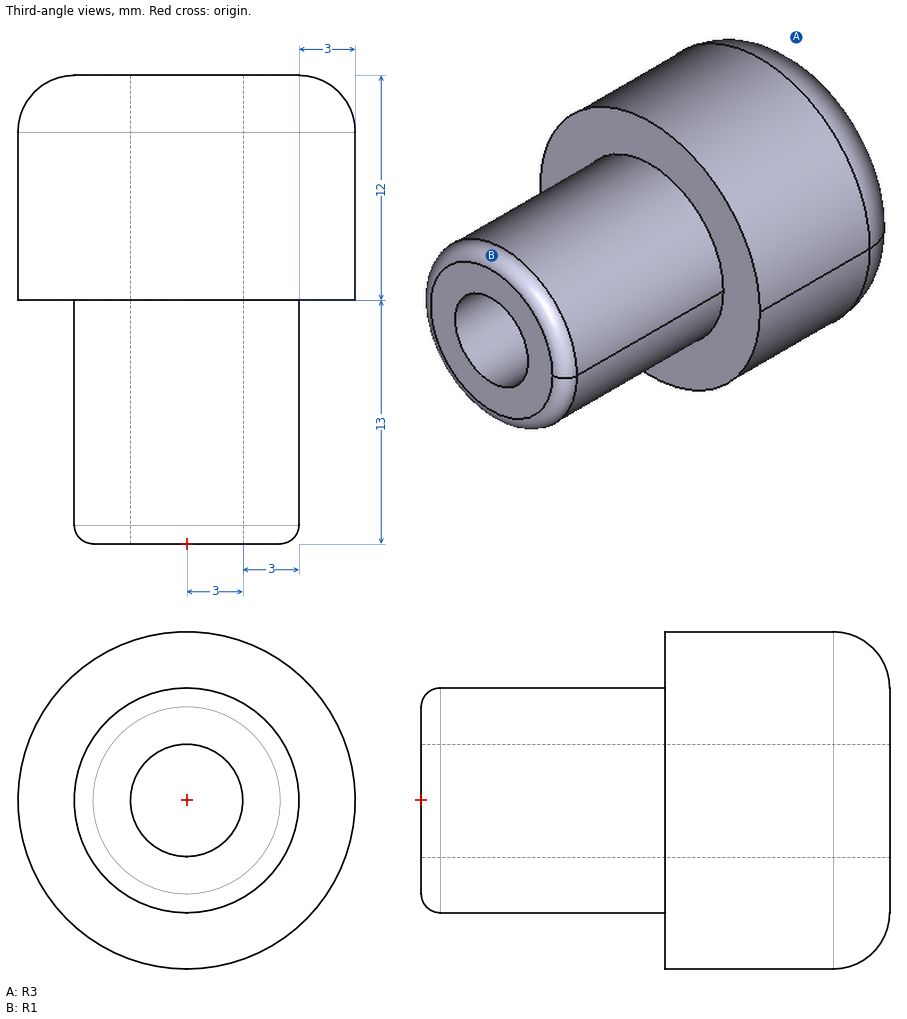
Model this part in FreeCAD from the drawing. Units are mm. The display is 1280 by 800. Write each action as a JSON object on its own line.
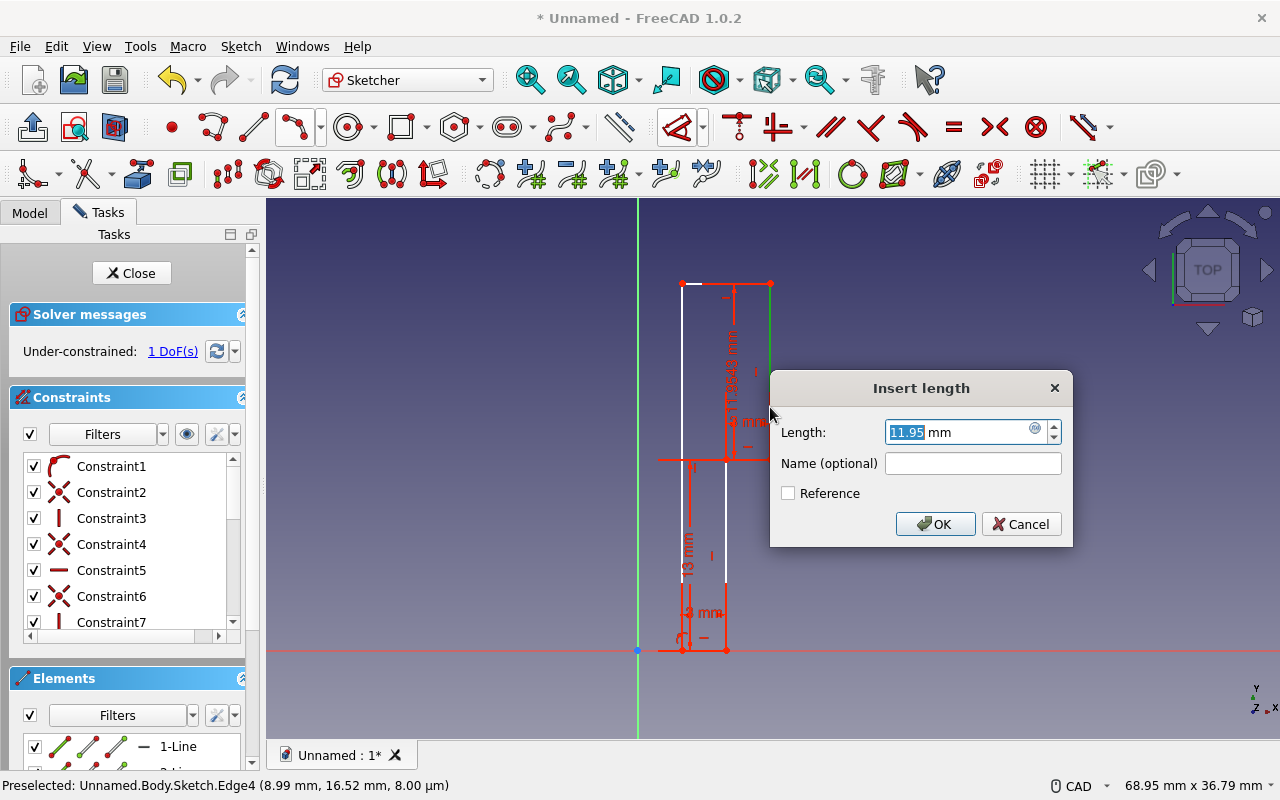
{"action": "type", "text": "12"}
{"action": "key", "text": "Return"}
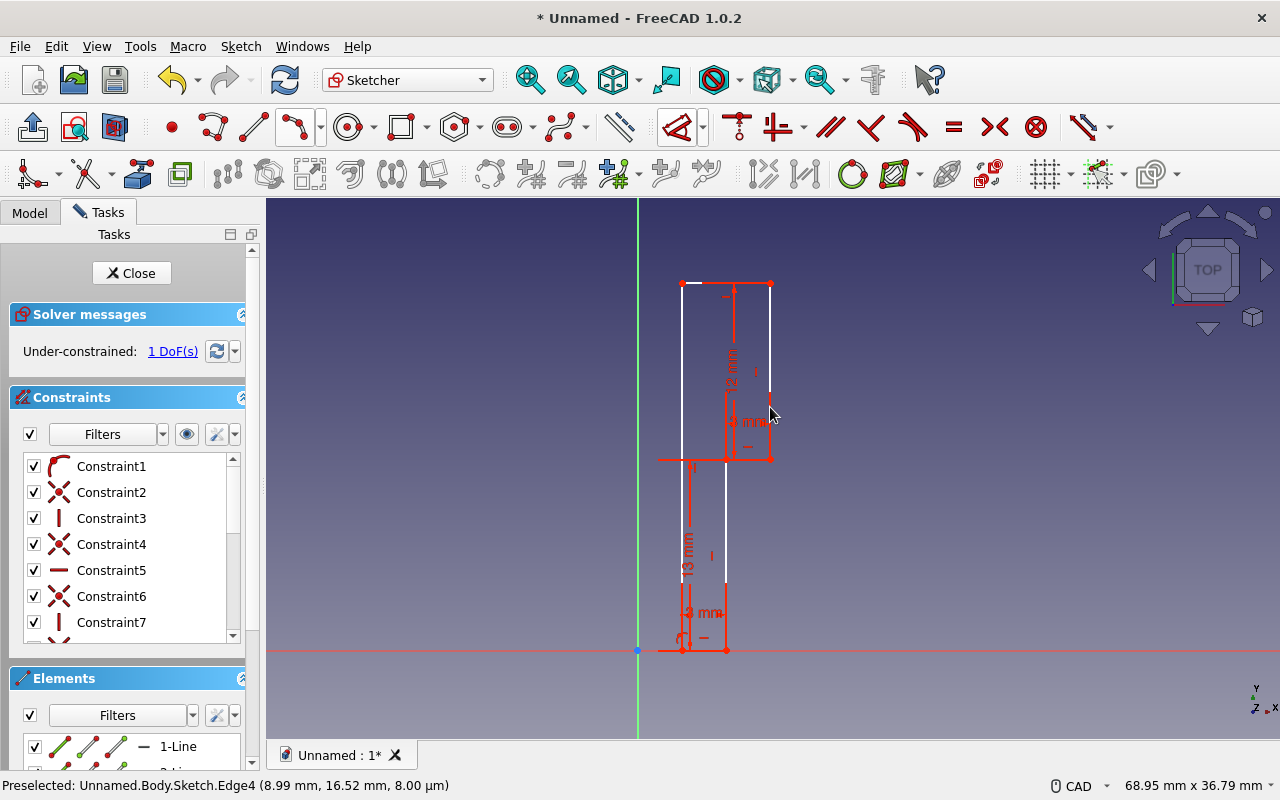
{"action": "left_click", "coordinate": [682, 651]}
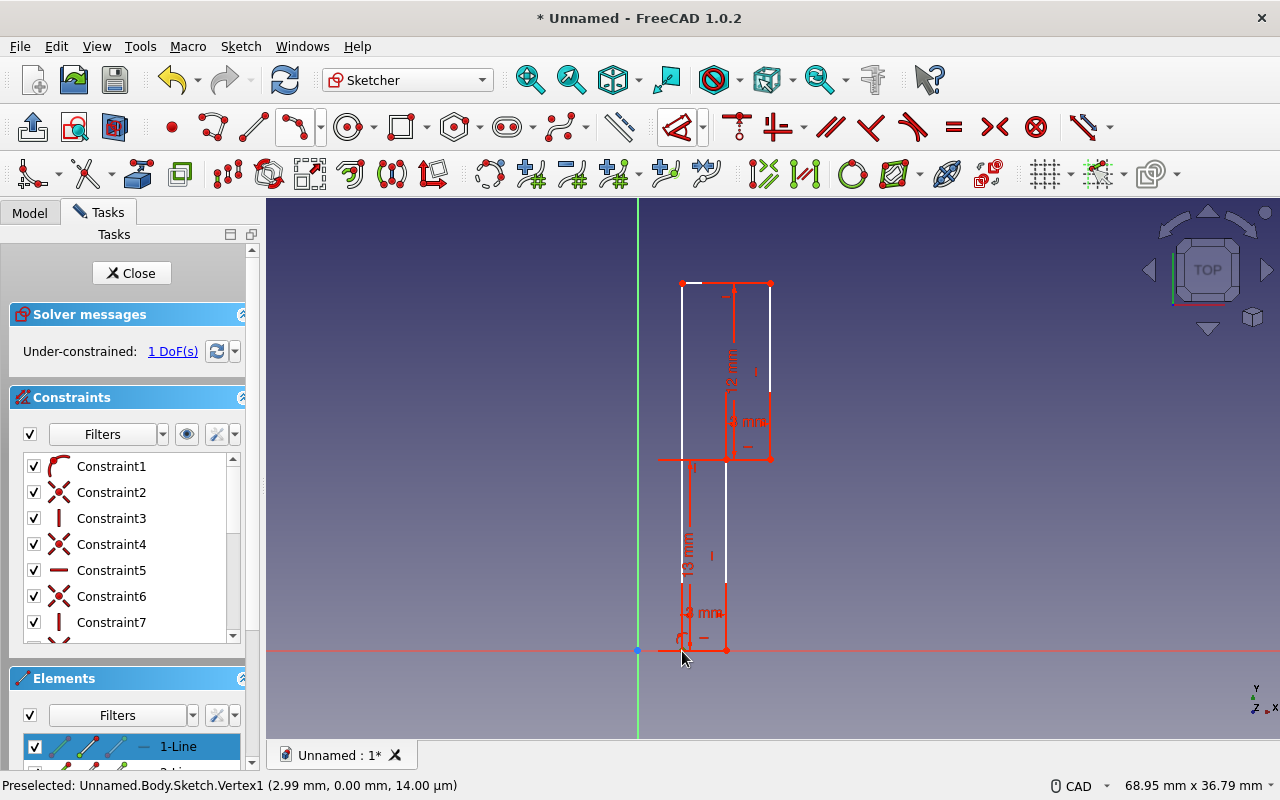
{"action": "key", "text": "l"}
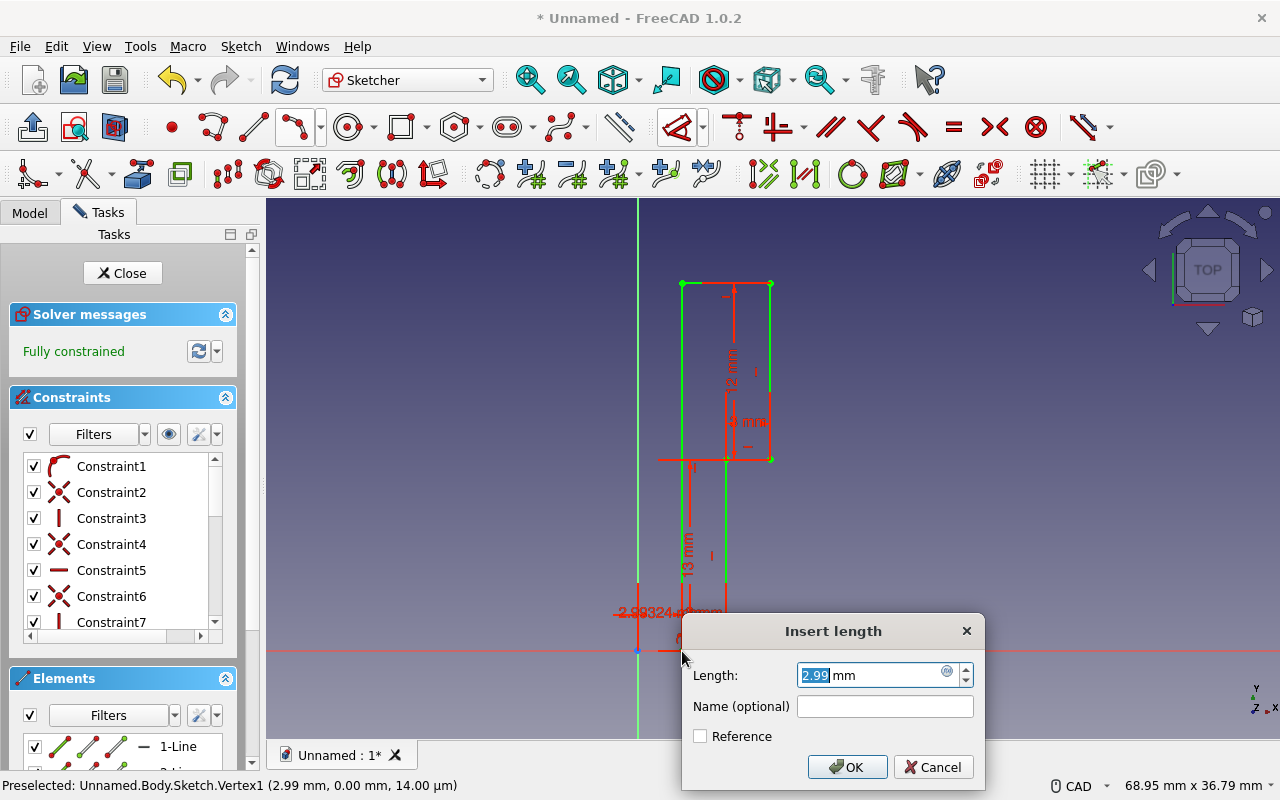
{"action": "type", "text": "3"}
{"action": "key", "text": "Return"}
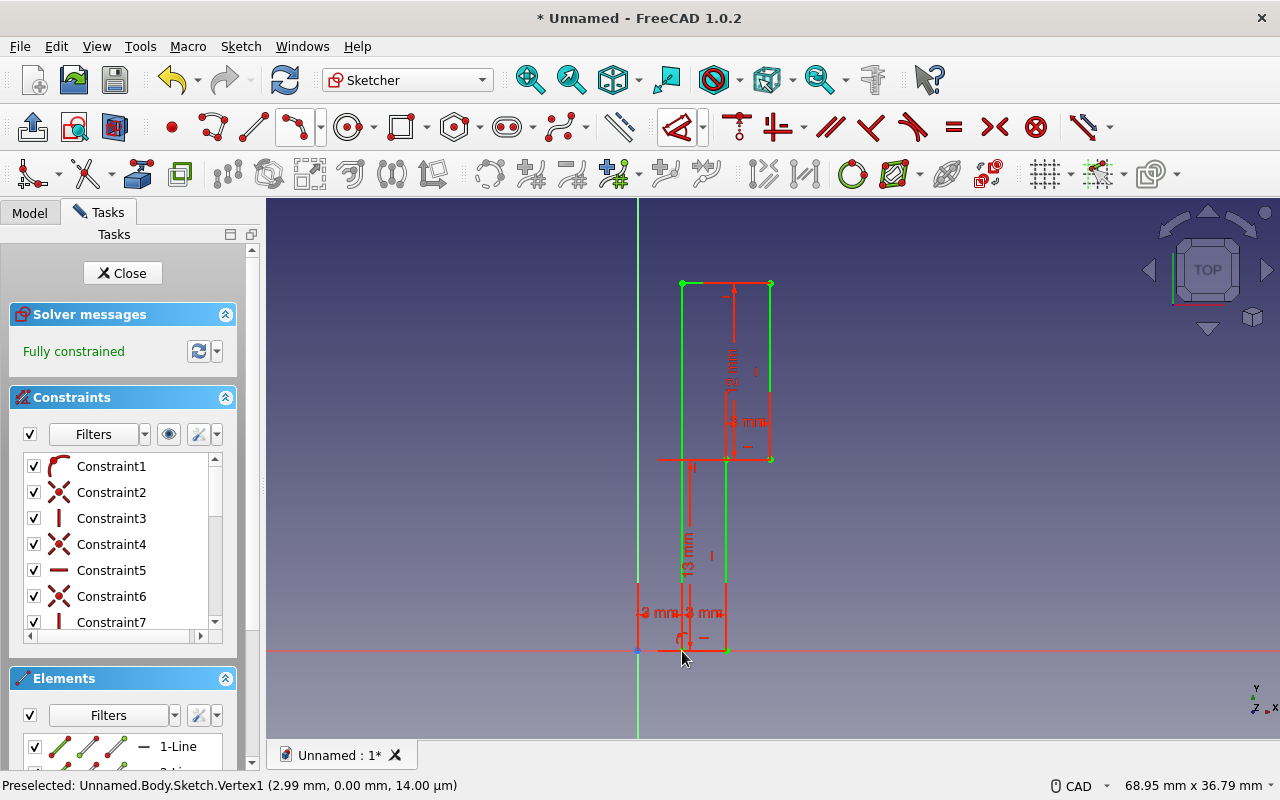
{"action": "left_click", "coordinate": [123, 273]}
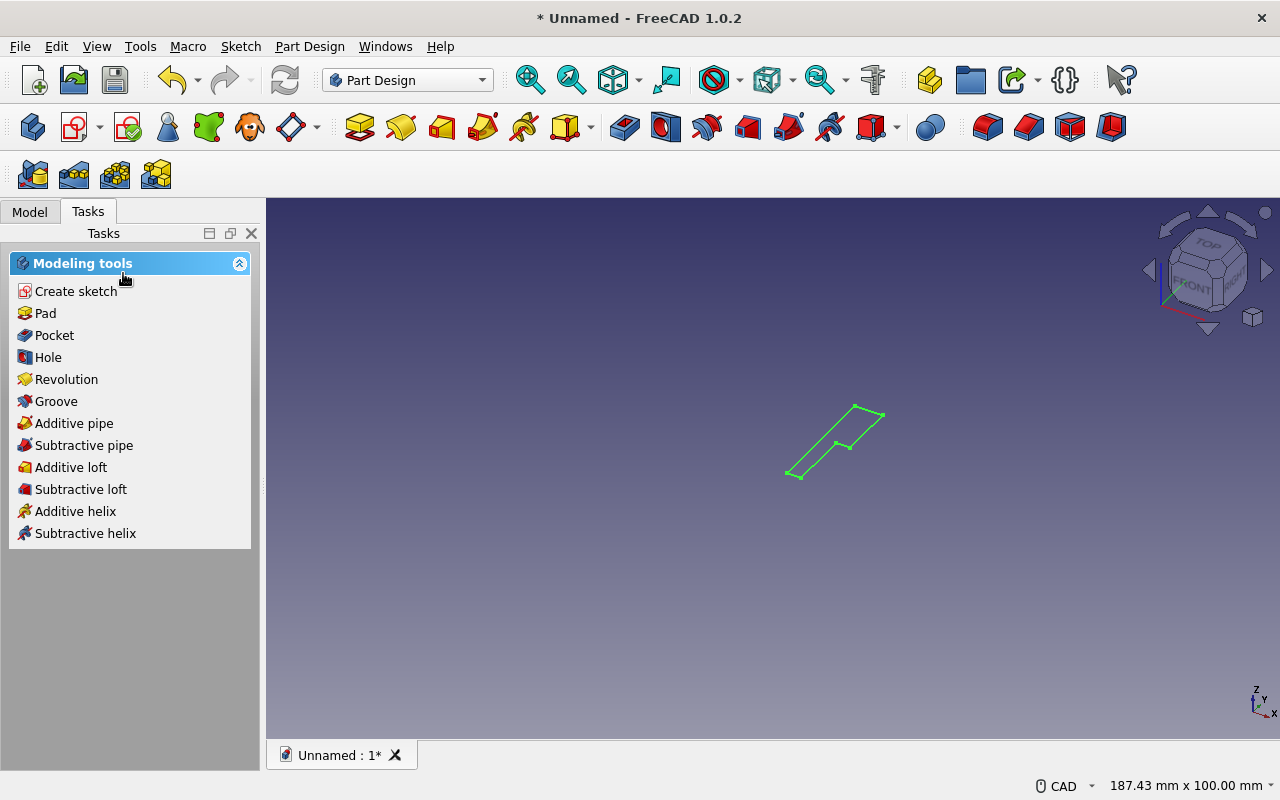
{"action": "left_click", "coordinate": [401, 128]}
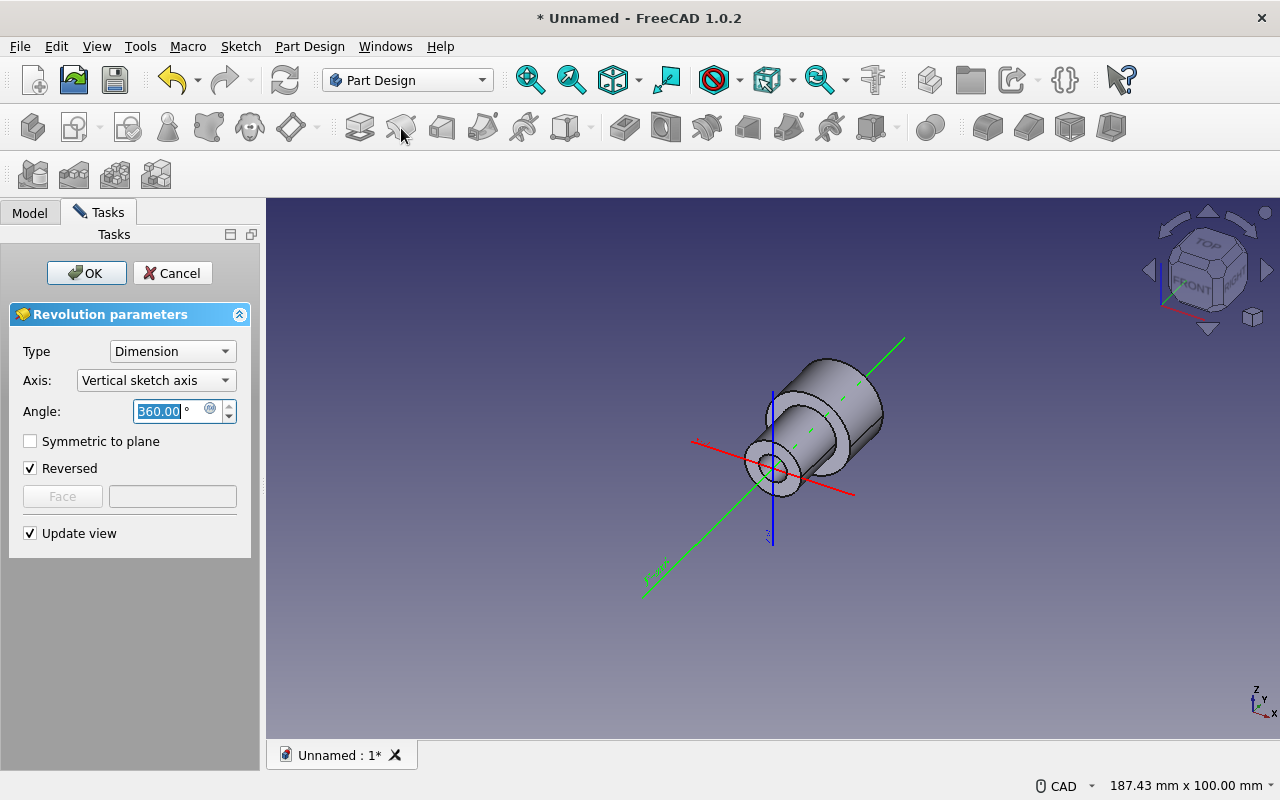
{"action": "left_click", "coordinate": [87, 273]}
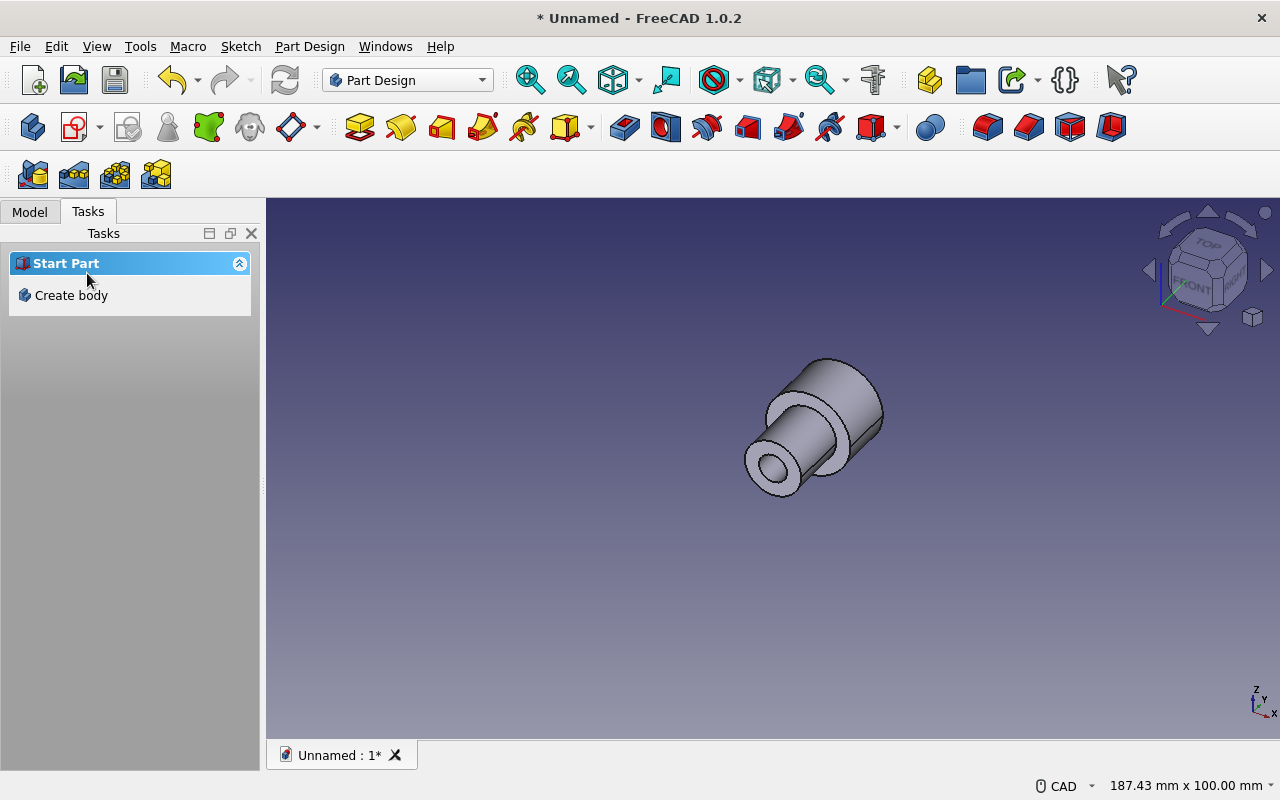
{"action": "key", "text": "v f"}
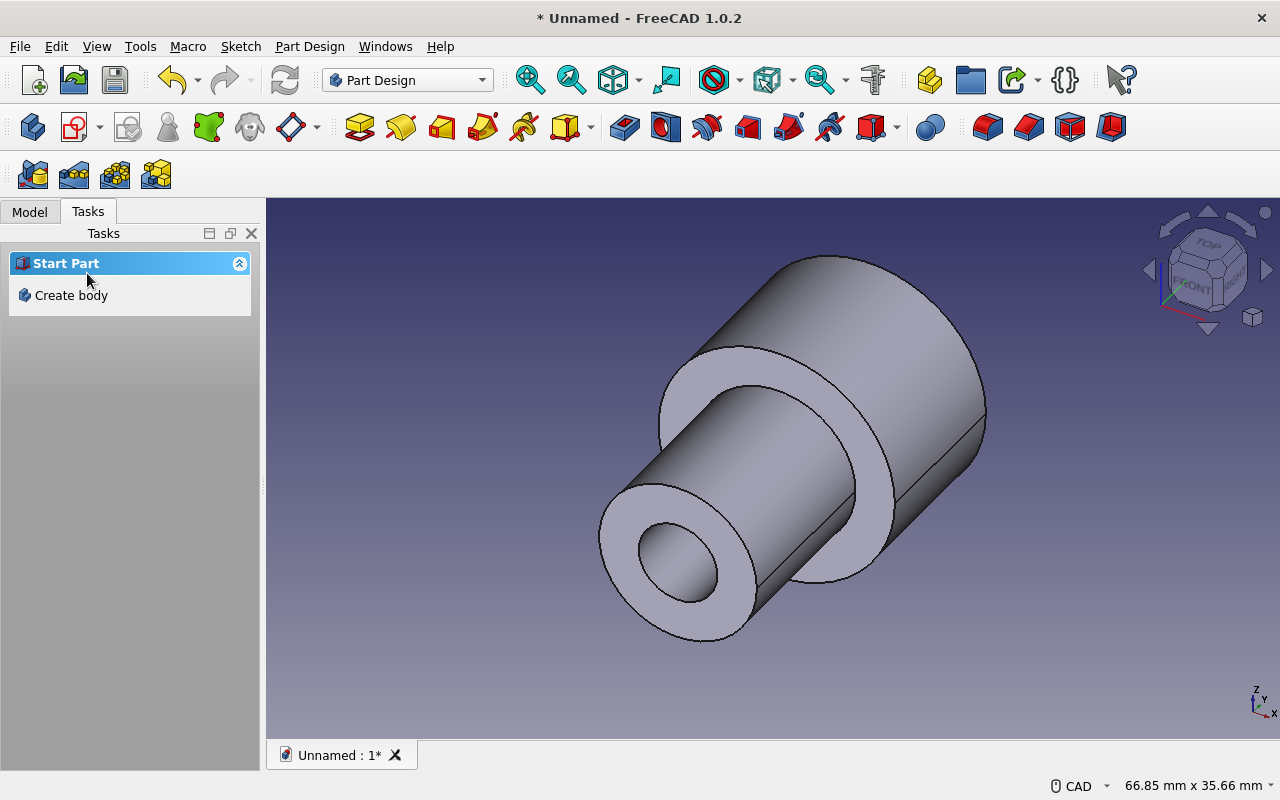
{"action": "key", "text": "0"}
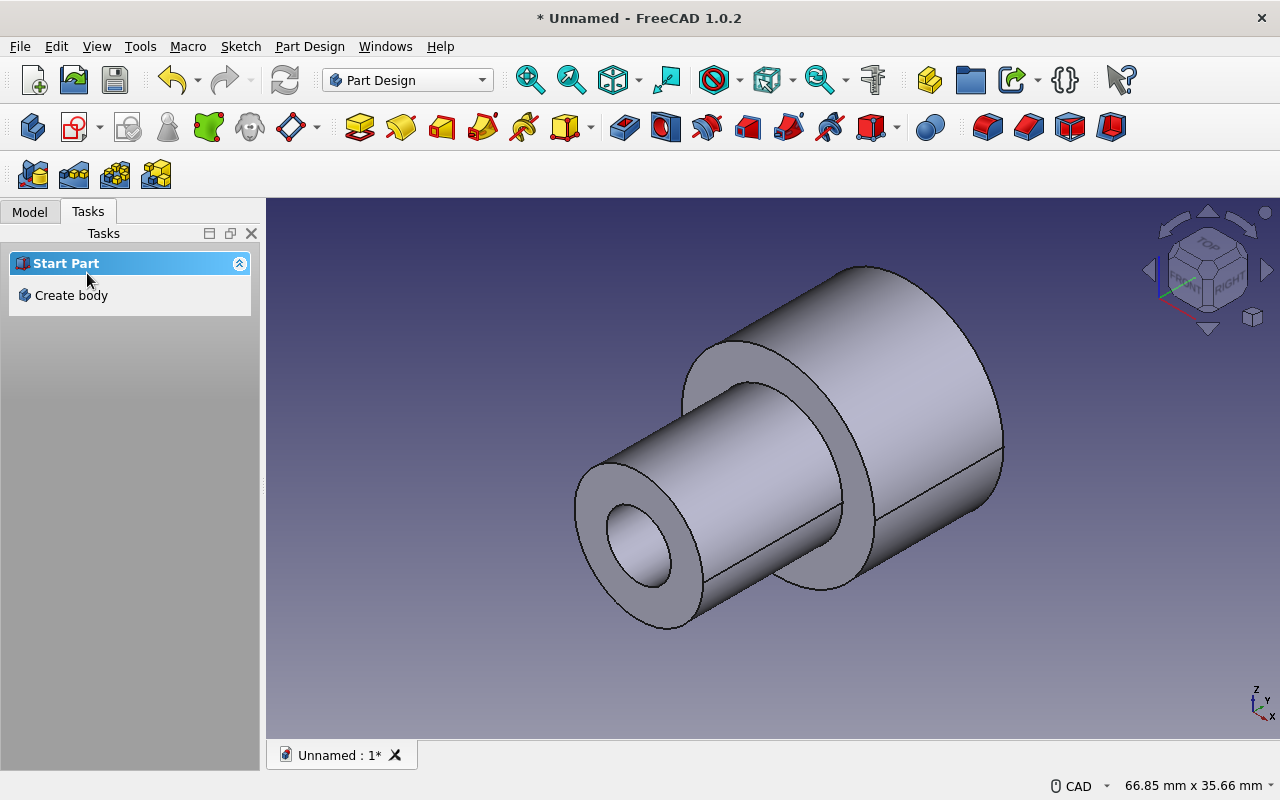
{"action": "key", "text": "2"}